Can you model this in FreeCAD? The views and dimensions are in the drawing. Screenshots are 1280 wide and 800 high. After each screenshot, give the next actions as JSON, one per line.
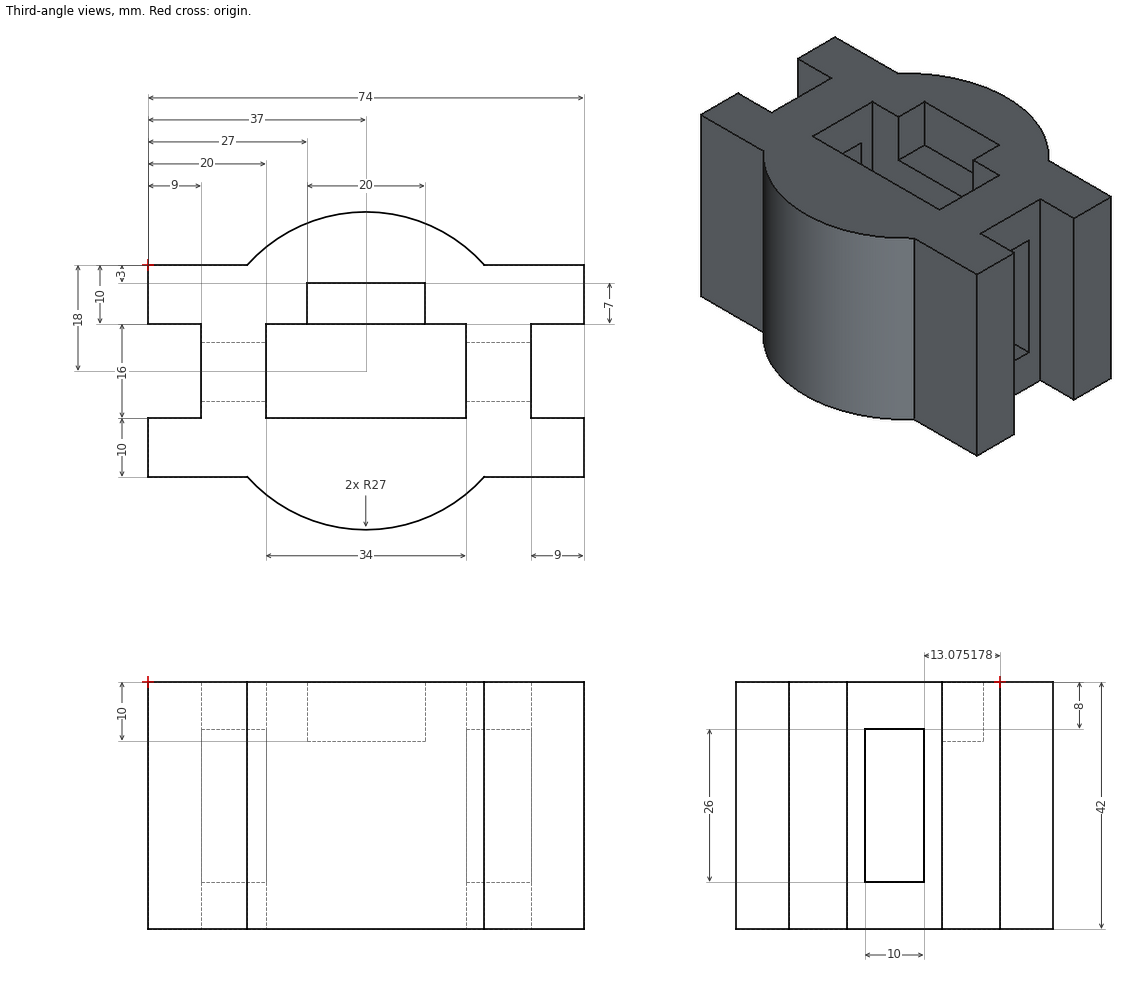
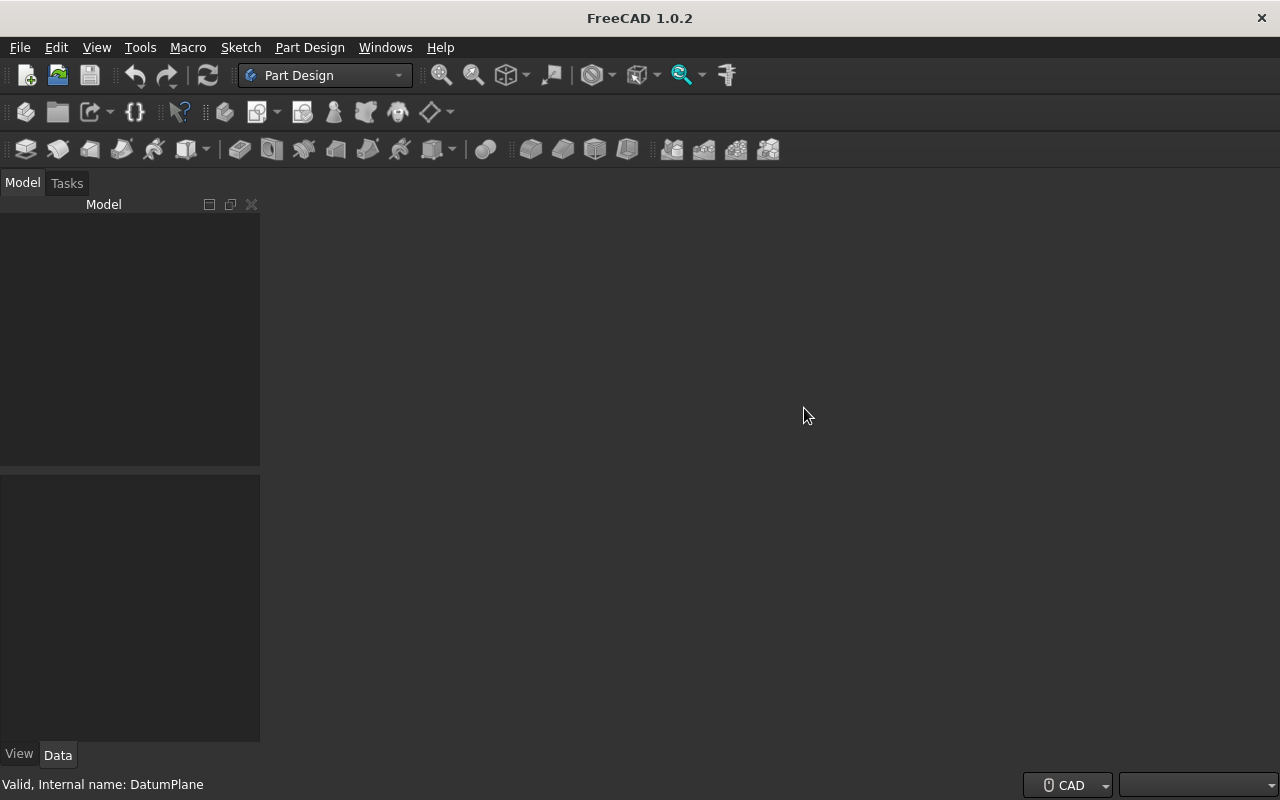
{"action": "left_click", "coordinate": [26, 76]}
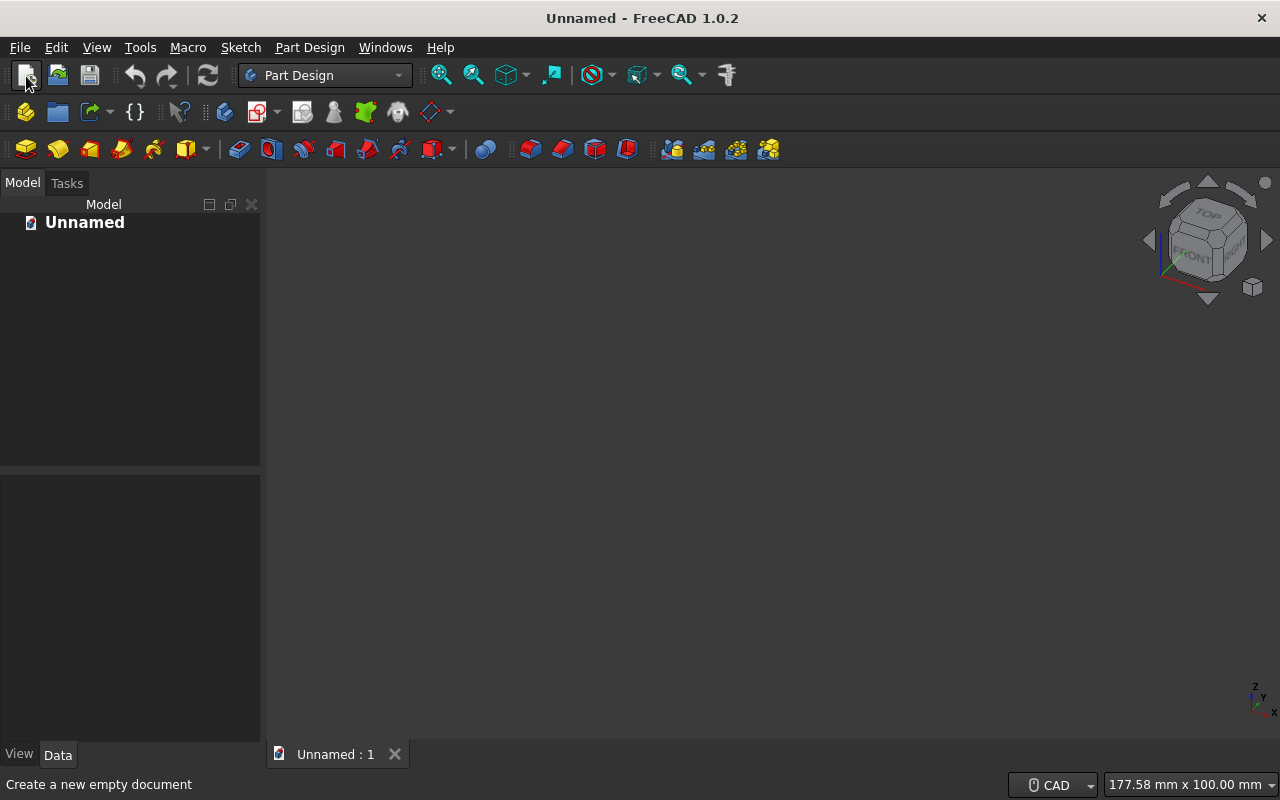
{"action": "left_click", "coordinate": [258, 112]}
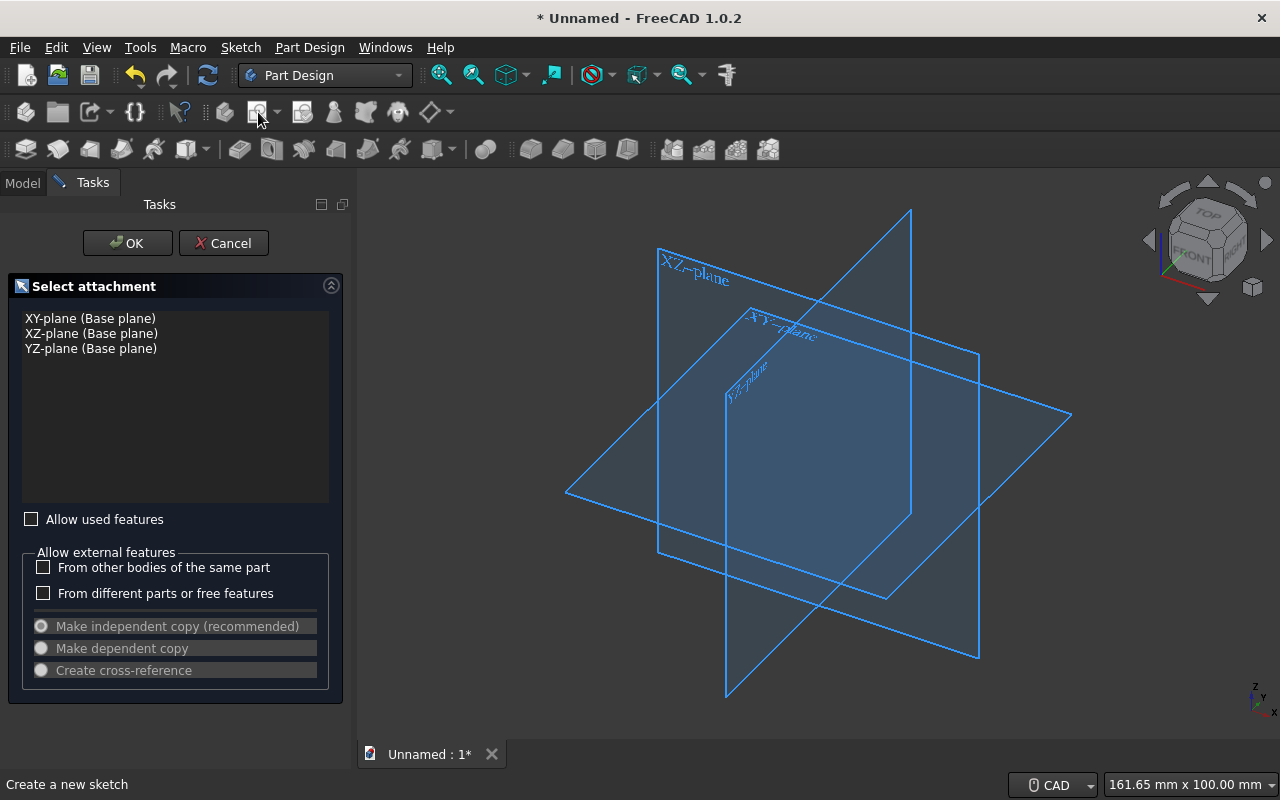
{"action": "left_click", "coordinate": [82, 318]}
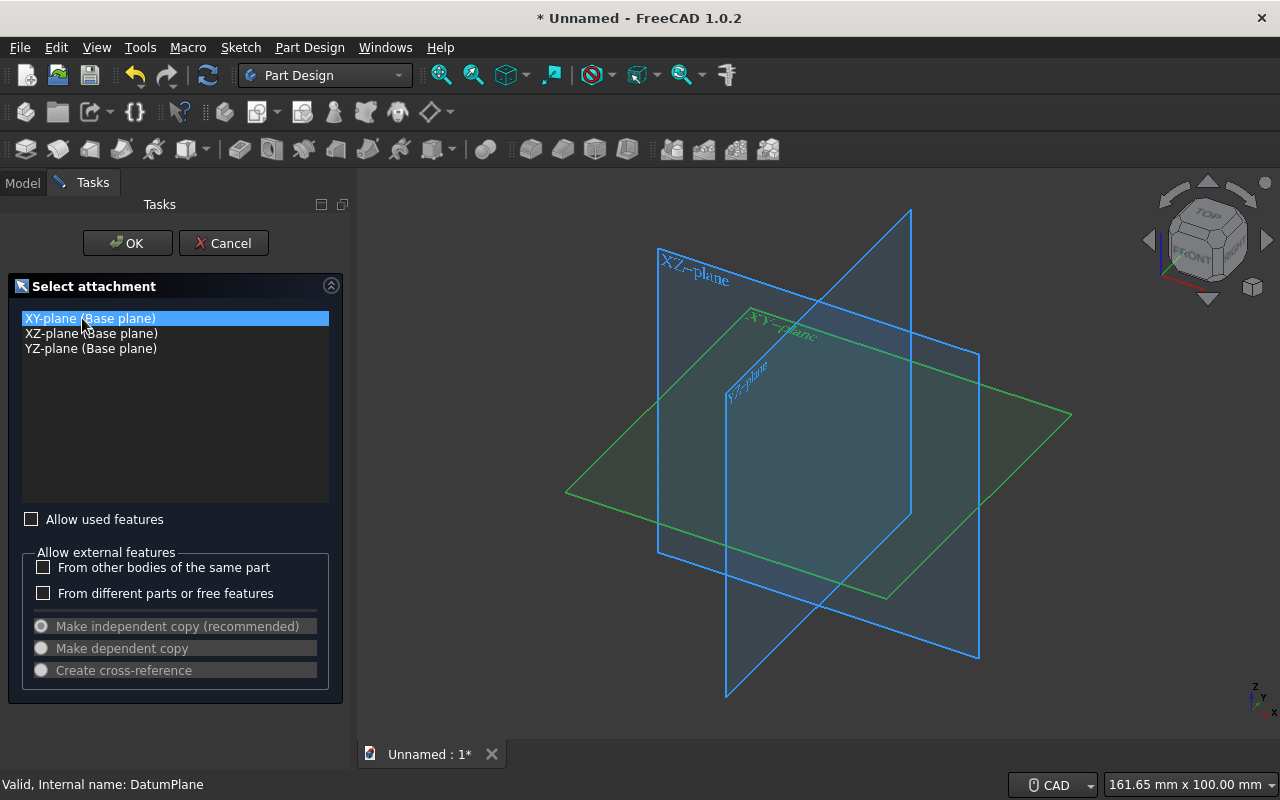
{"action": "left_click", "coordinate": [128, 243]}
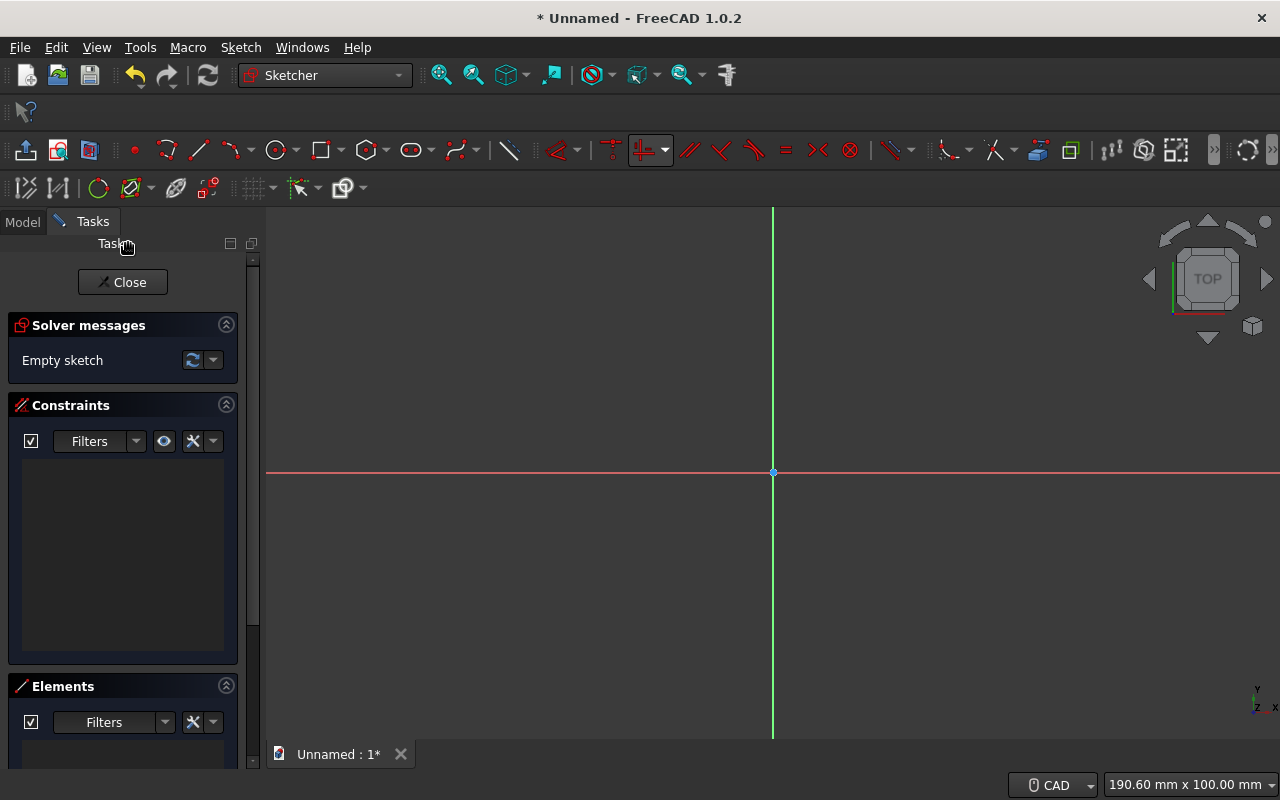
{"action": "scroll", "coordinate": [294, 235], "scroll_direction": "down", "scroll_amount": 1}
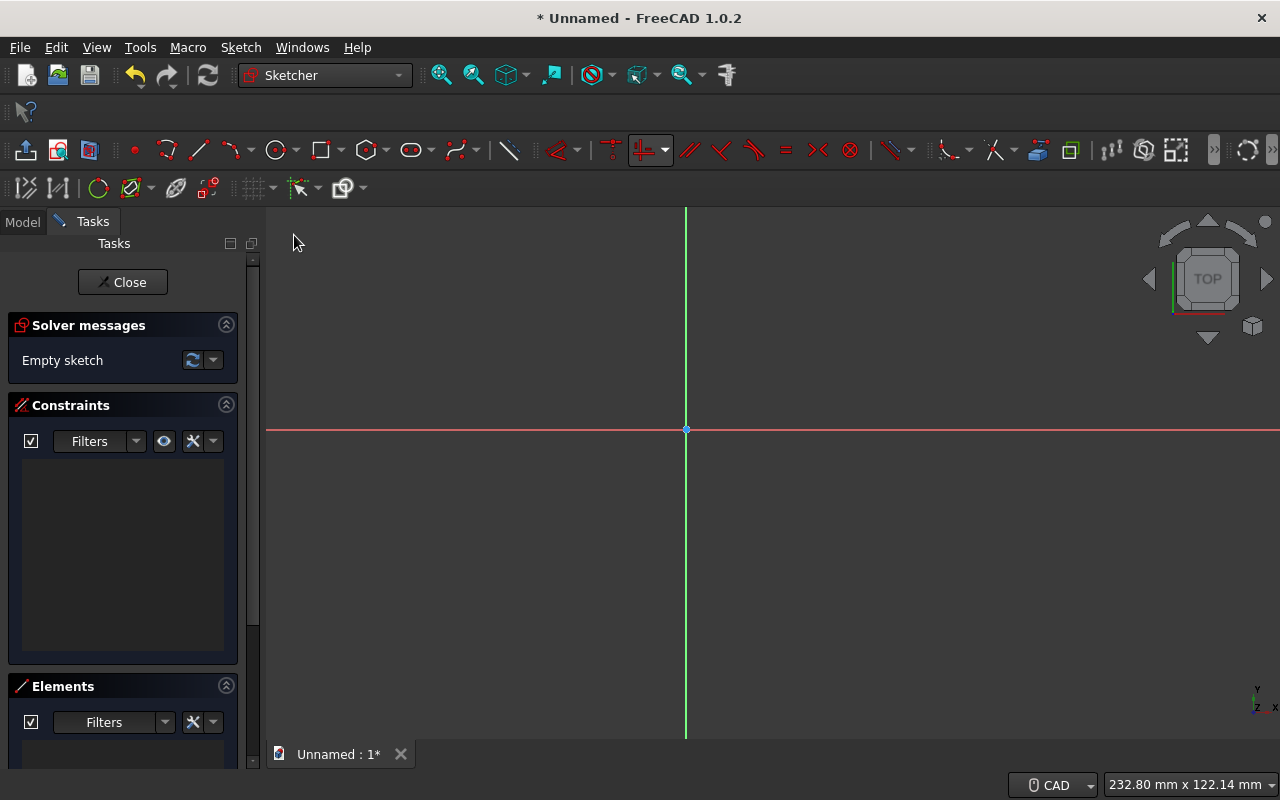
{"action": "scroll", "coordinate": [1115, 580], "scroll_direction": "up", "scroll_amount": 2}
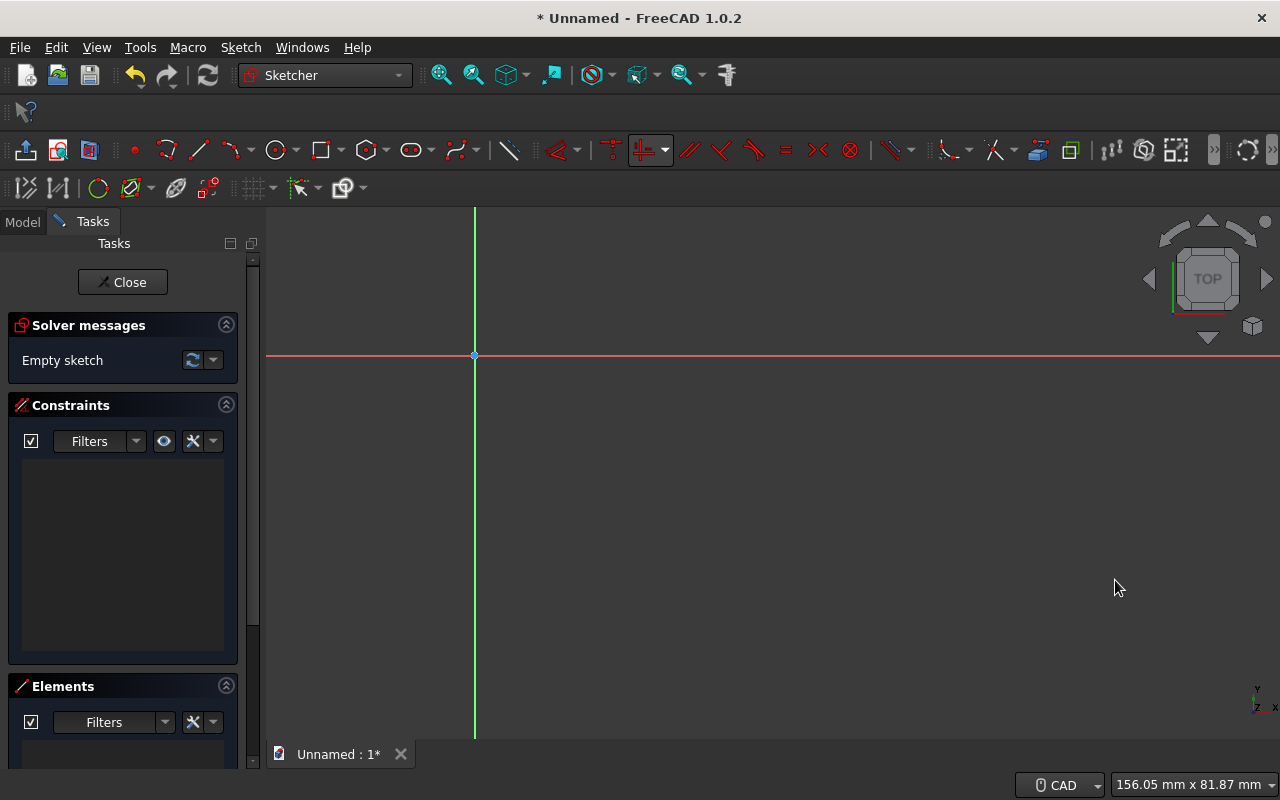
{"action": "left_click", "coordinate": [168, 150]}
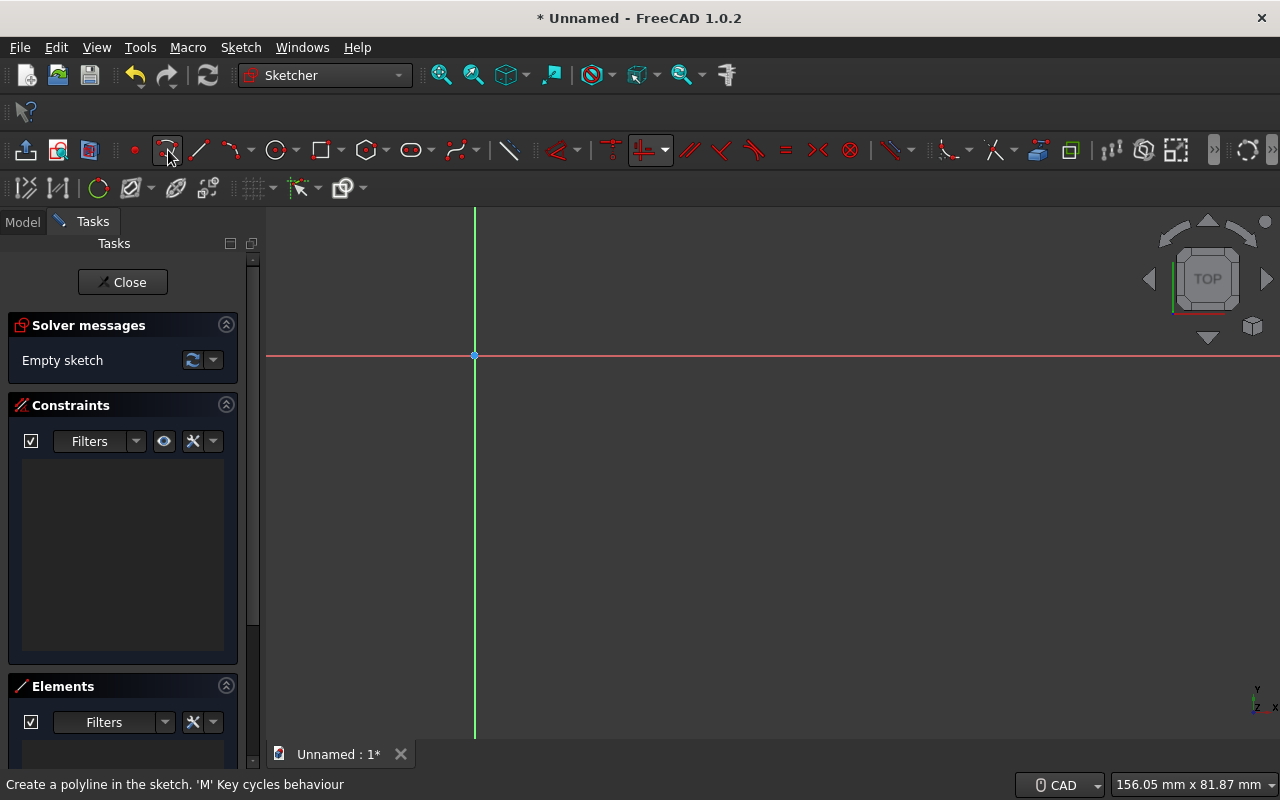
{"action": "left_click", "coordinate": [585, 356]}
{"action": "left_click", "coordinate": [475, 356]}
{"action": "left_click", "coordinate": [484, 421]}
{"action": "left_click", "coordinate": [533, 421]}
{"action": "left_click", "coordinate": [533, 525]}
{"action": "left_click", "coordinate": [475, 525]}
{"action": "left_click", "coordinate": [484, 590]}
{"action": "left_click", "coordinate": [585, 590]}
{"action": "right_click", "coordinate": [585, 590]}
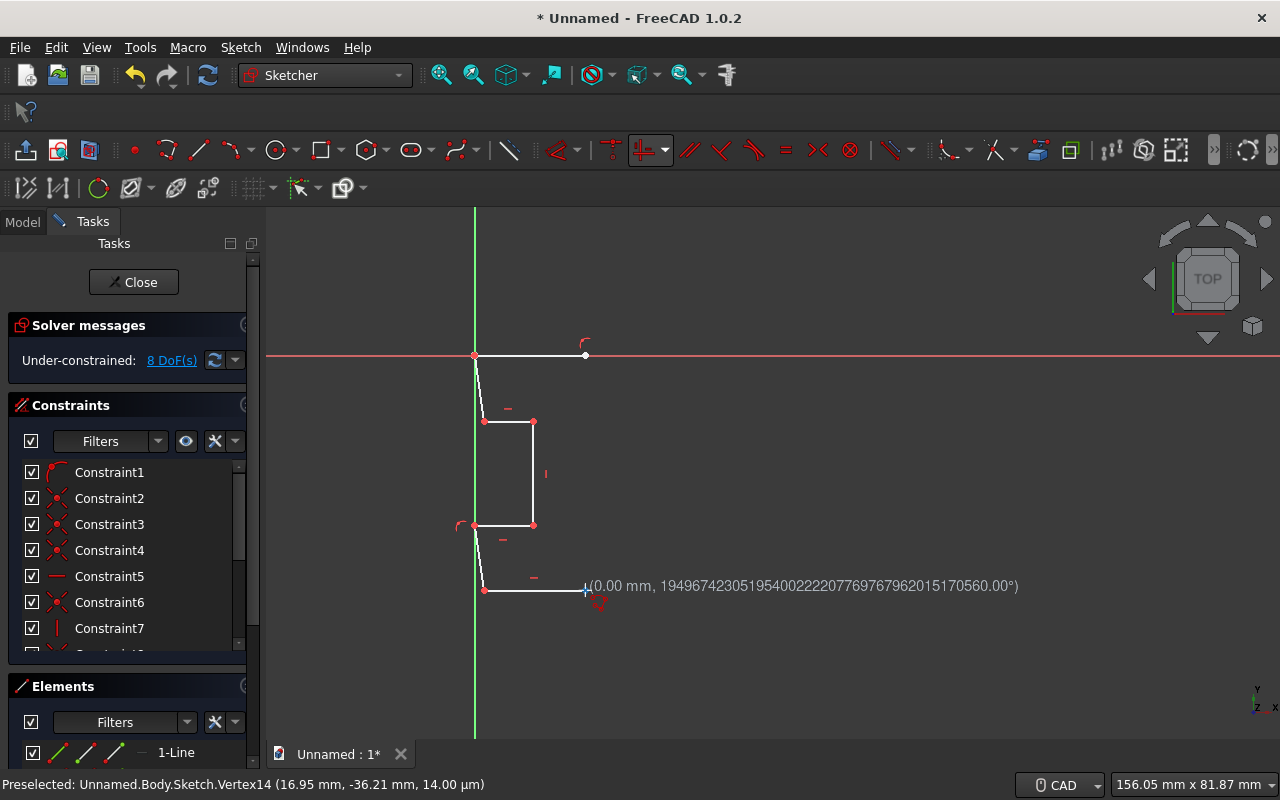
{"action": "left_click", "coordinate": [846, 590]}
{"action": "left_click", "coordinate": [956, 590]}
{"action": "left_click", "coordinate": [956, 525]}
{"action": "left_click", "coordinate": [897, 525]}
{"action": "left_click", "coordinate": [897, 421]}
{"action": "left_click", "coordinate": [956, 421]}
{"action": "left_click", "coordinate": [956, 356]}
{"action": "left_click", "coordinate": [846, 365]}
{"action": "right_click", "coordinate": [846, 365]}